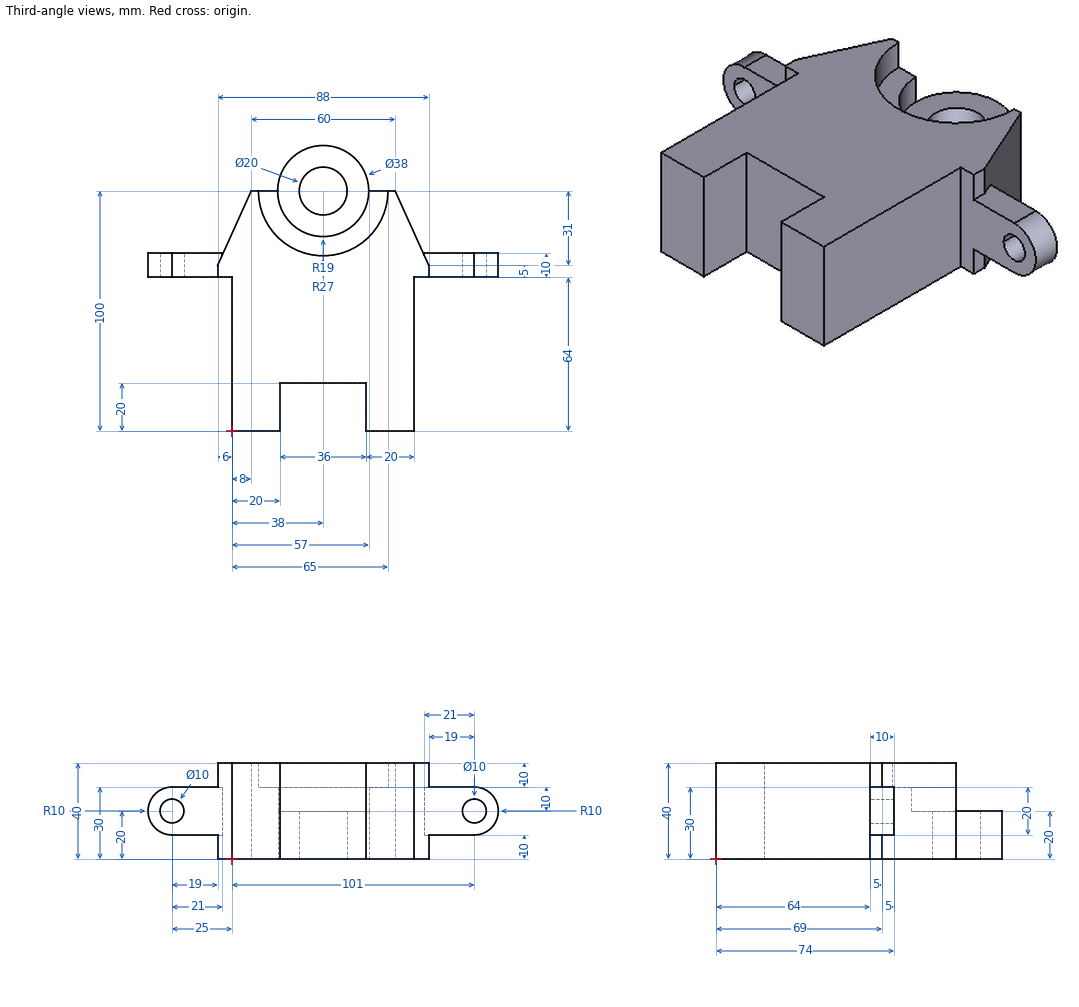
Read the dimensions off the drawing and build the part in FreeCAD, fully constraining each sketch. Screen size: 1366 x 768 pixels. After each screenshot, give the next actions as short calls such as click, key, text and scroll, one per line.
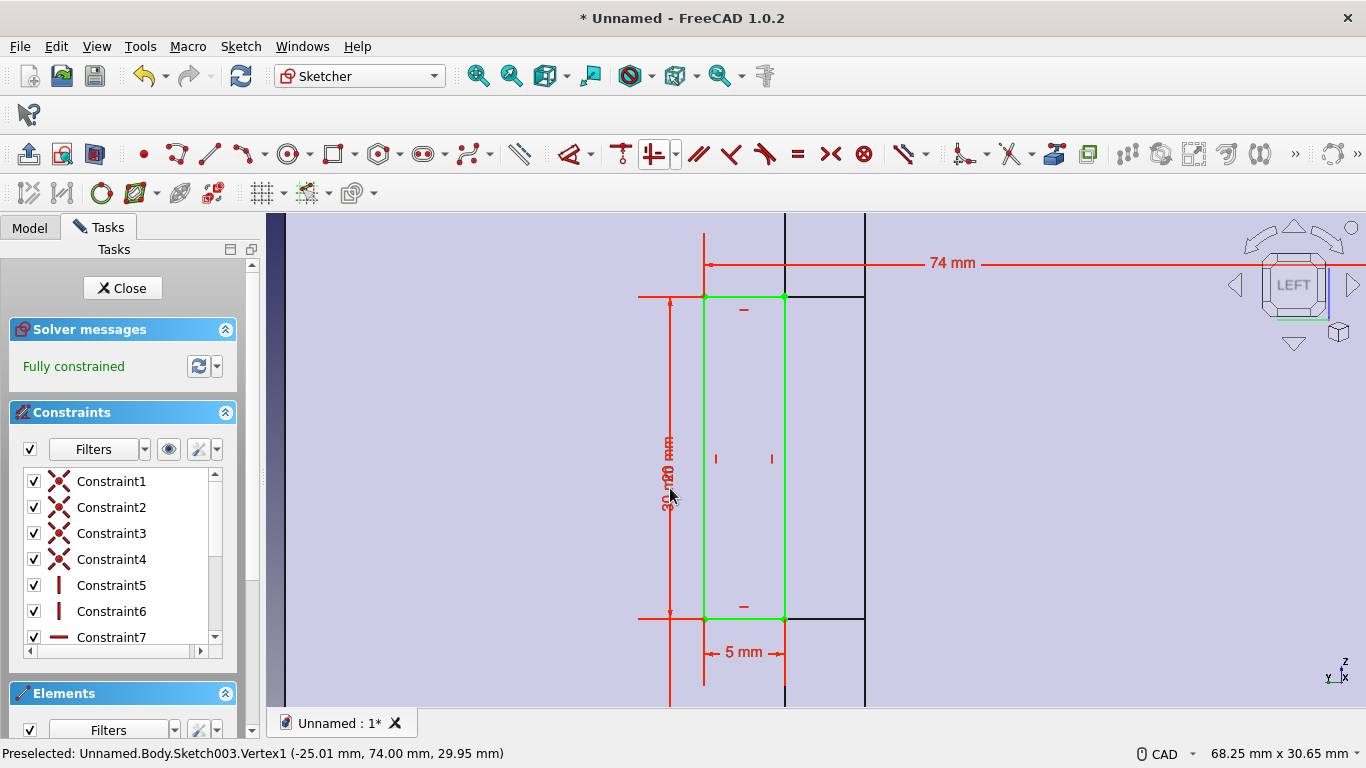
click(123, 288)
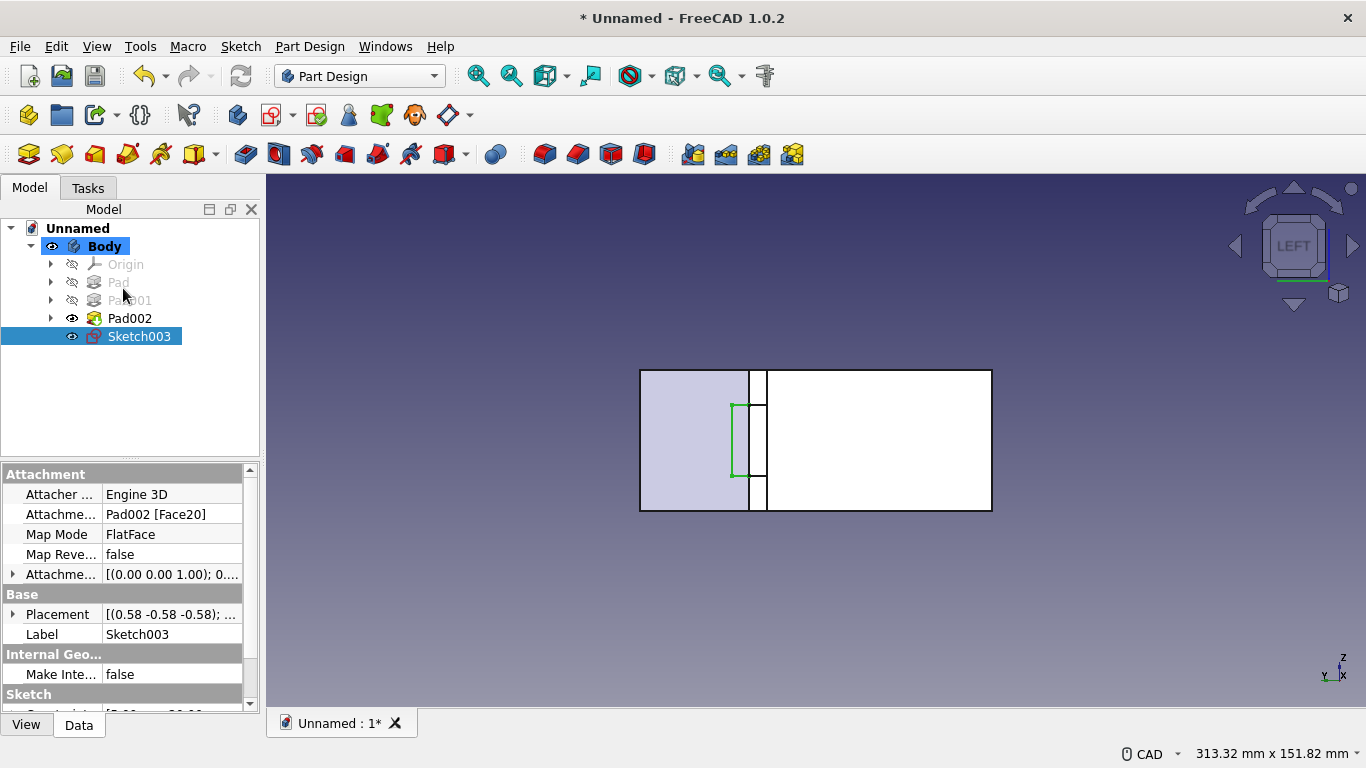
click(29, 154)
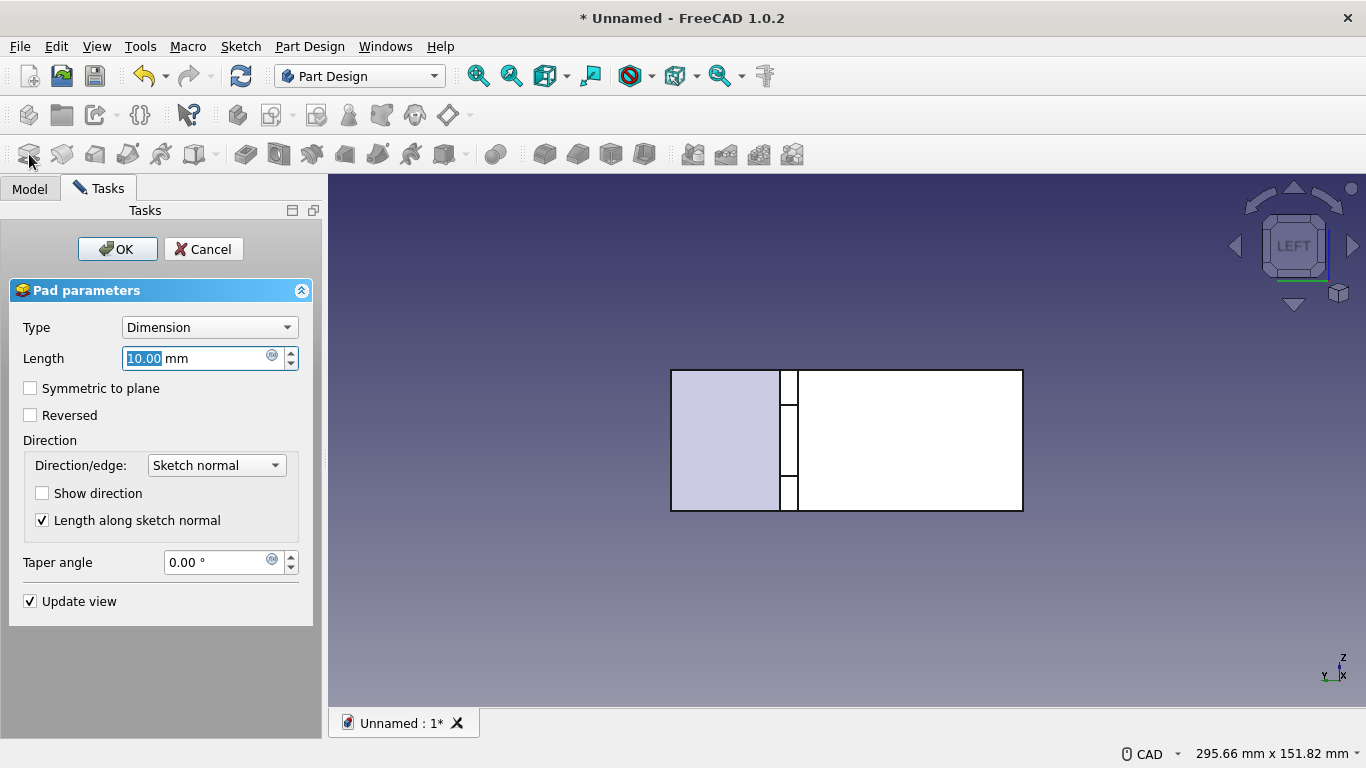
text(21)
key(Tab)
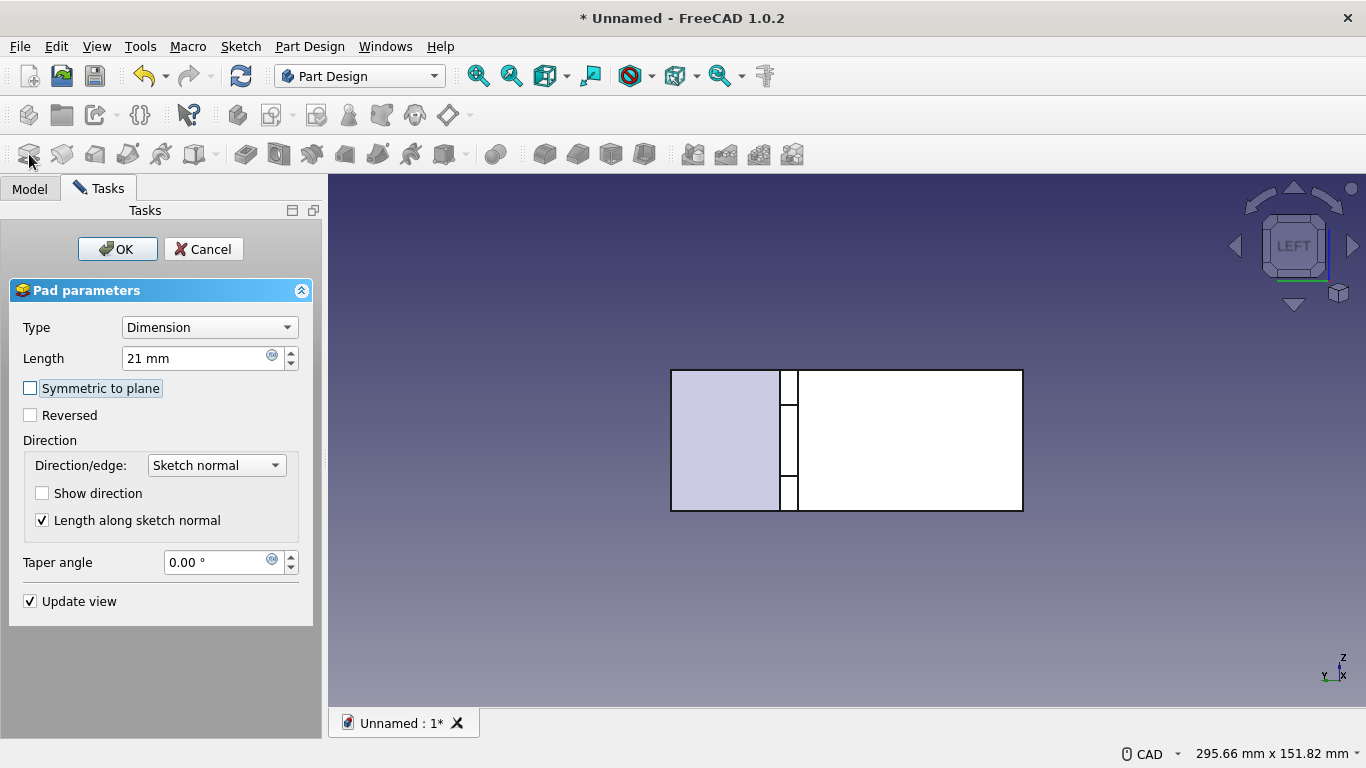
click(31, 415)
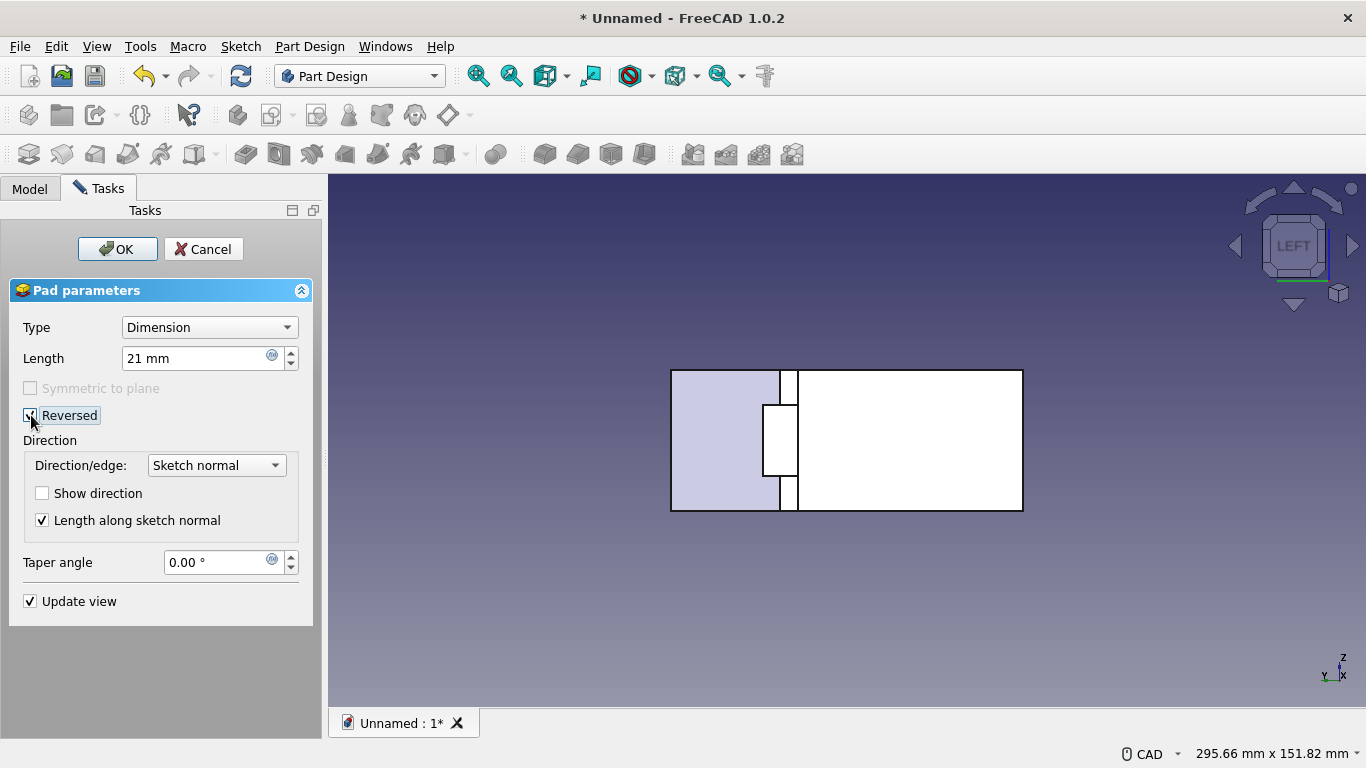
click(118, 249)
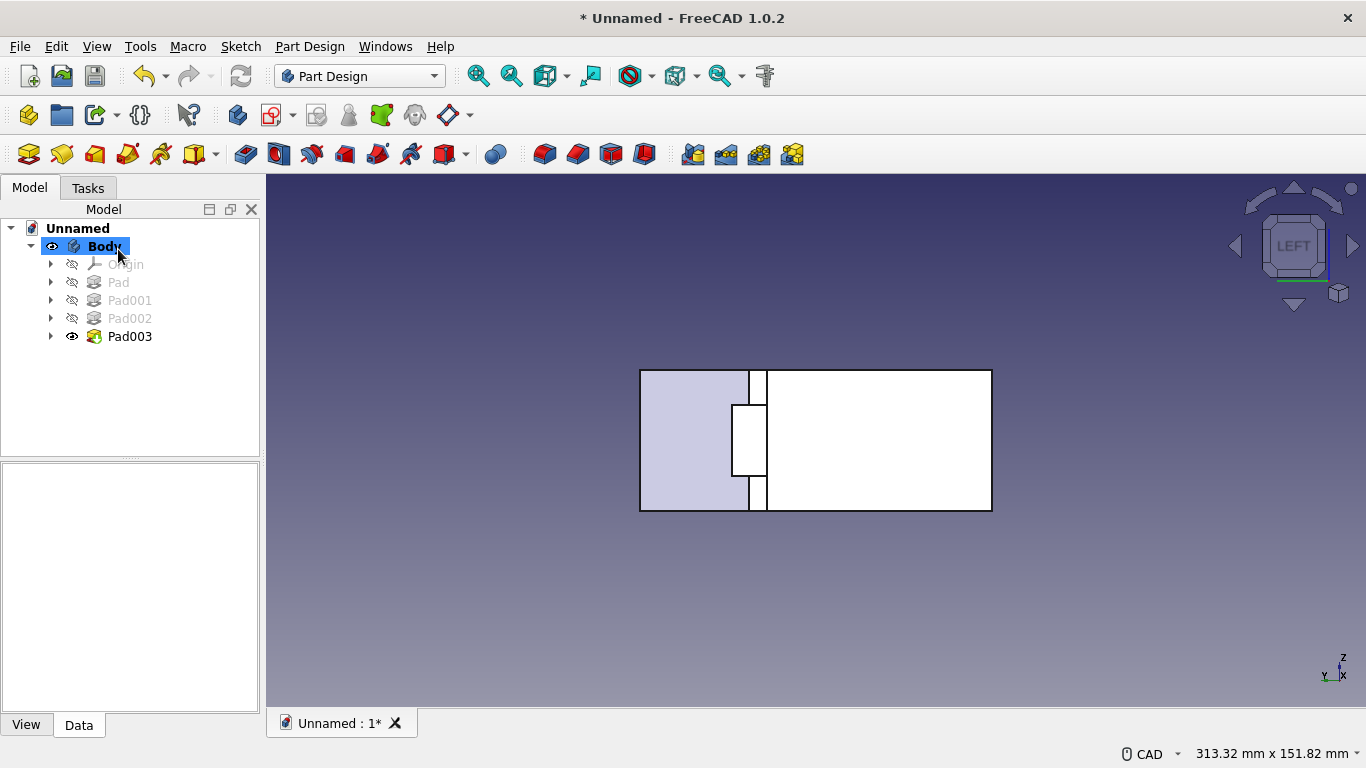
click(479, 76)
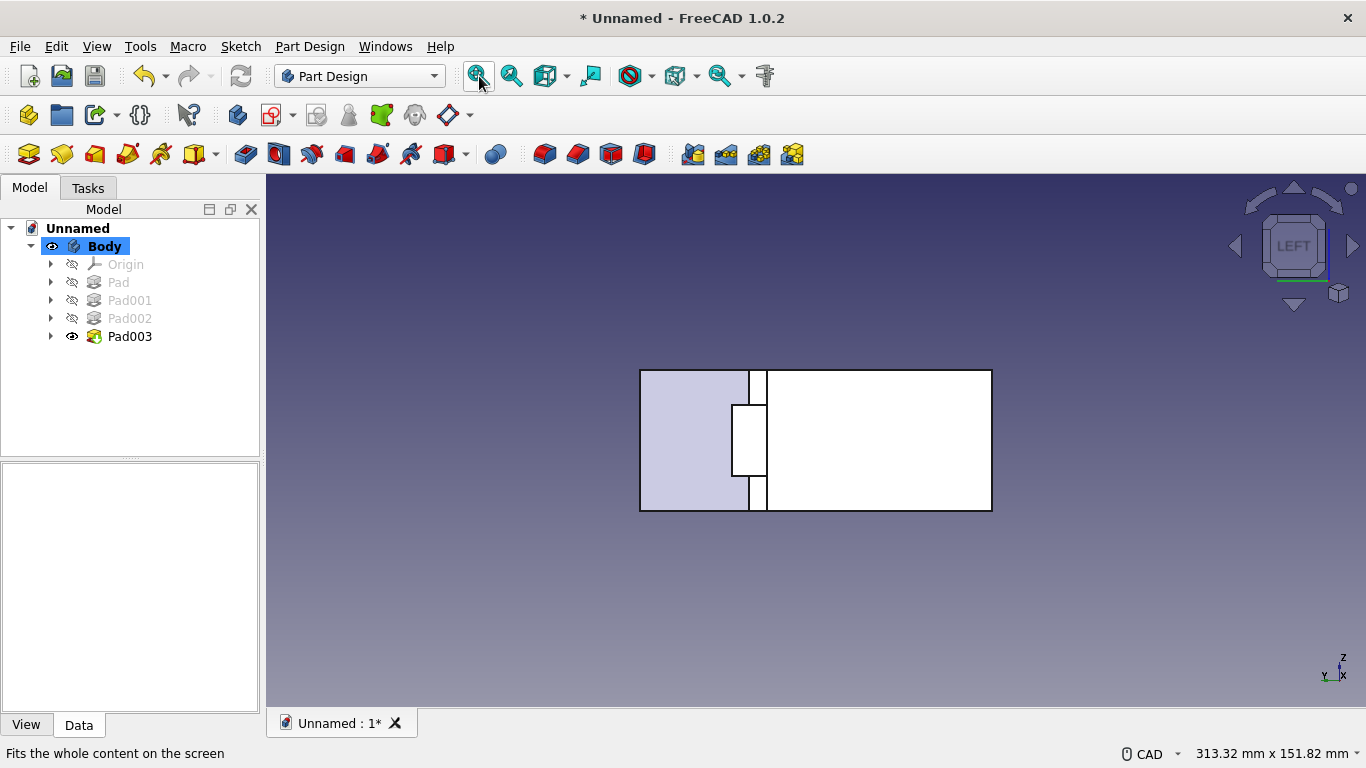
key(4)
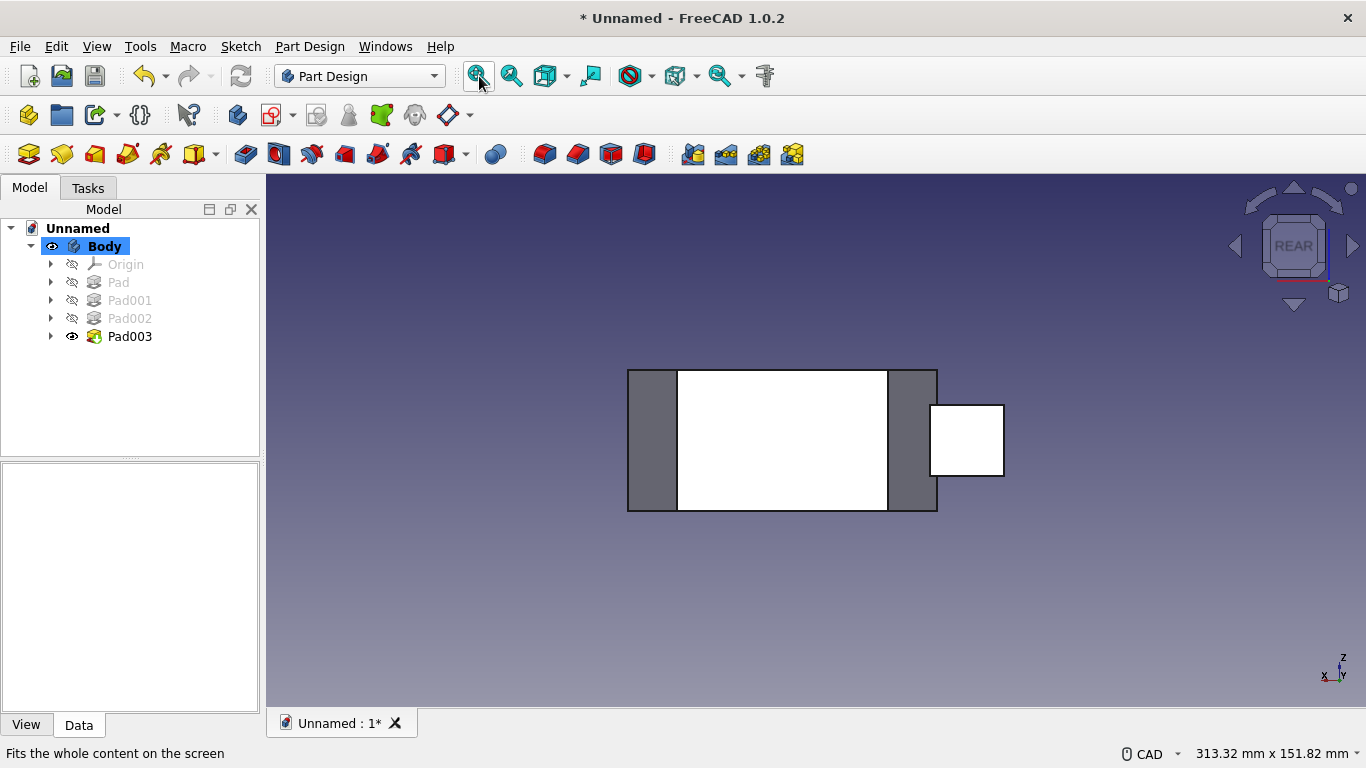
click(479, 76)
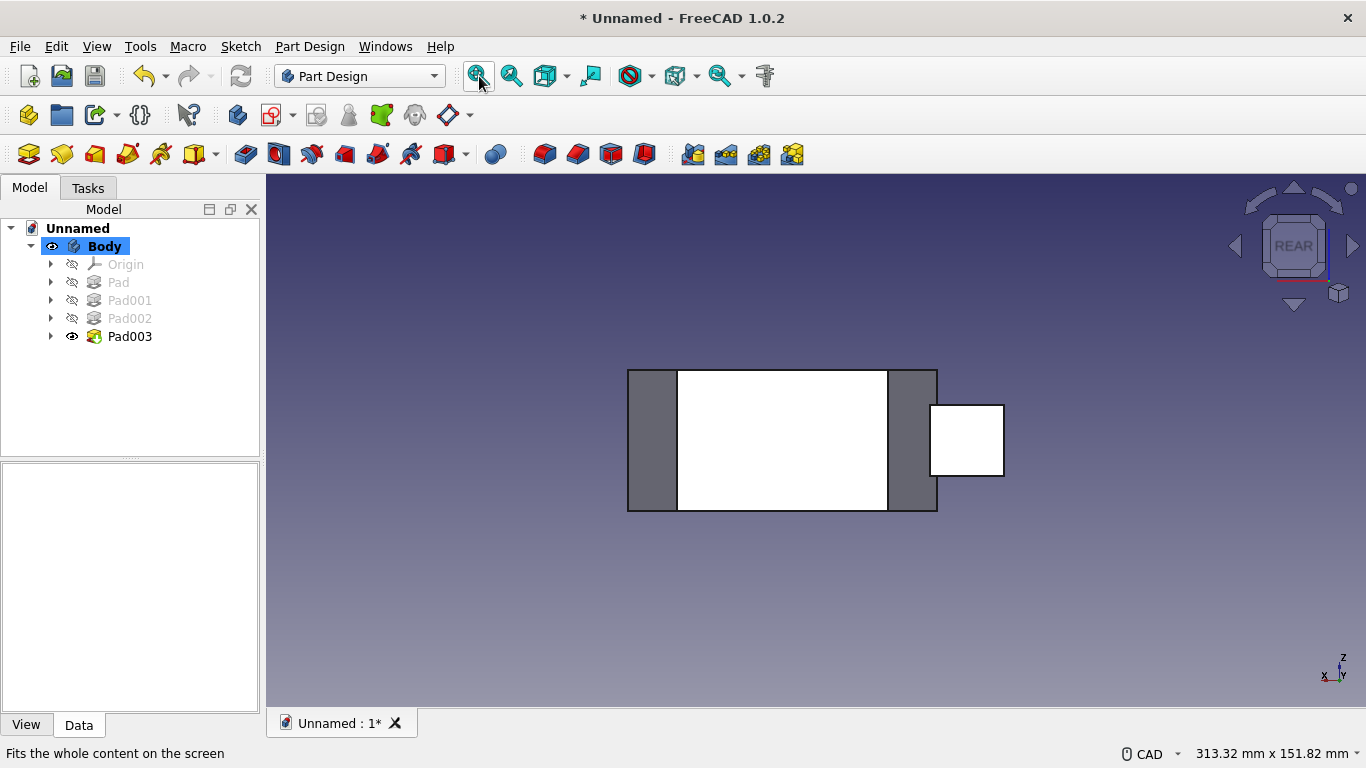
click(967, 440)